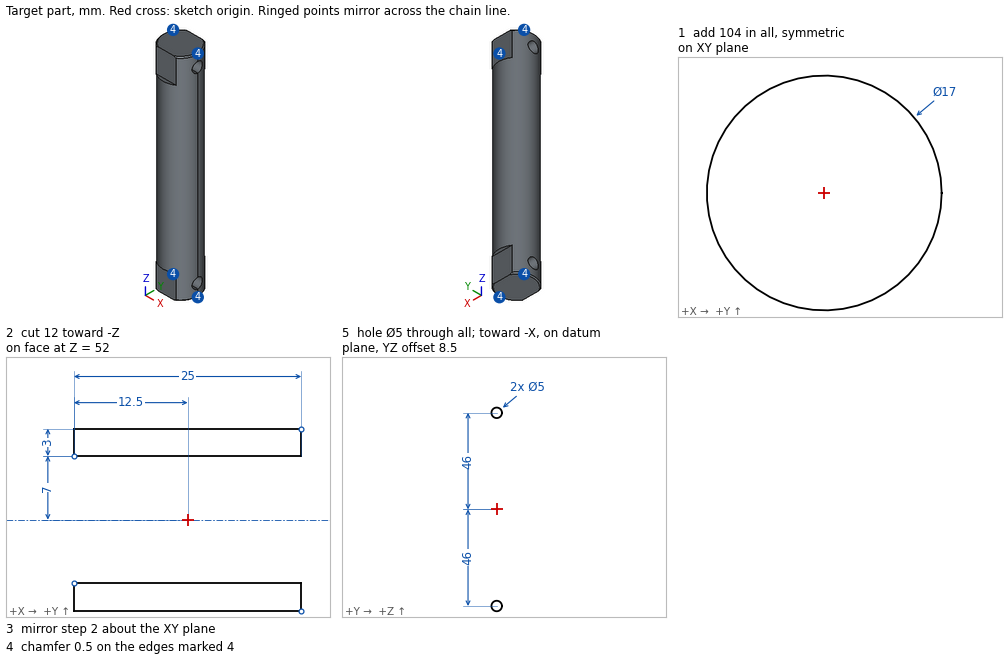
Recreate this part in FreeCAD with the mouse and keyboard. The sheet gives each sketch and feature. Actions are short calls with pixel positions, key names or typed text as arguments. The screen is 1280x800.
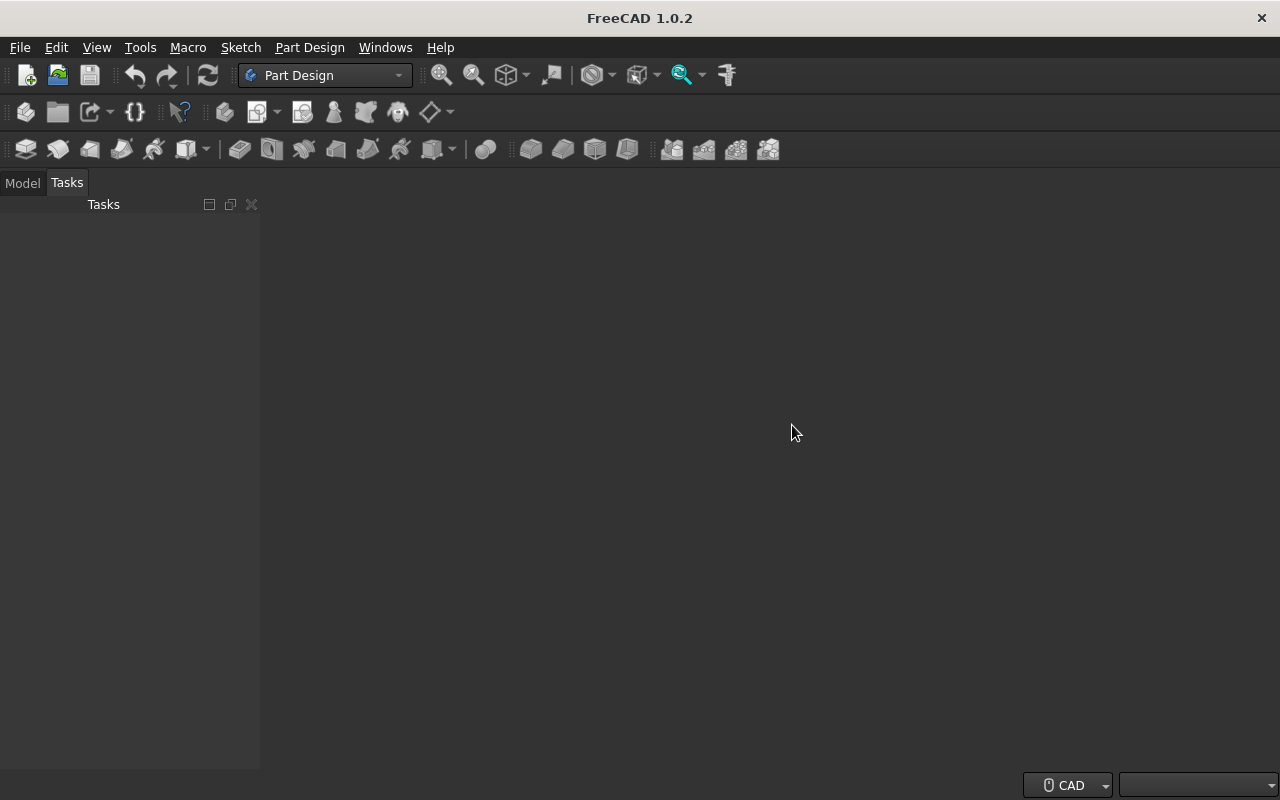
click(26, 76)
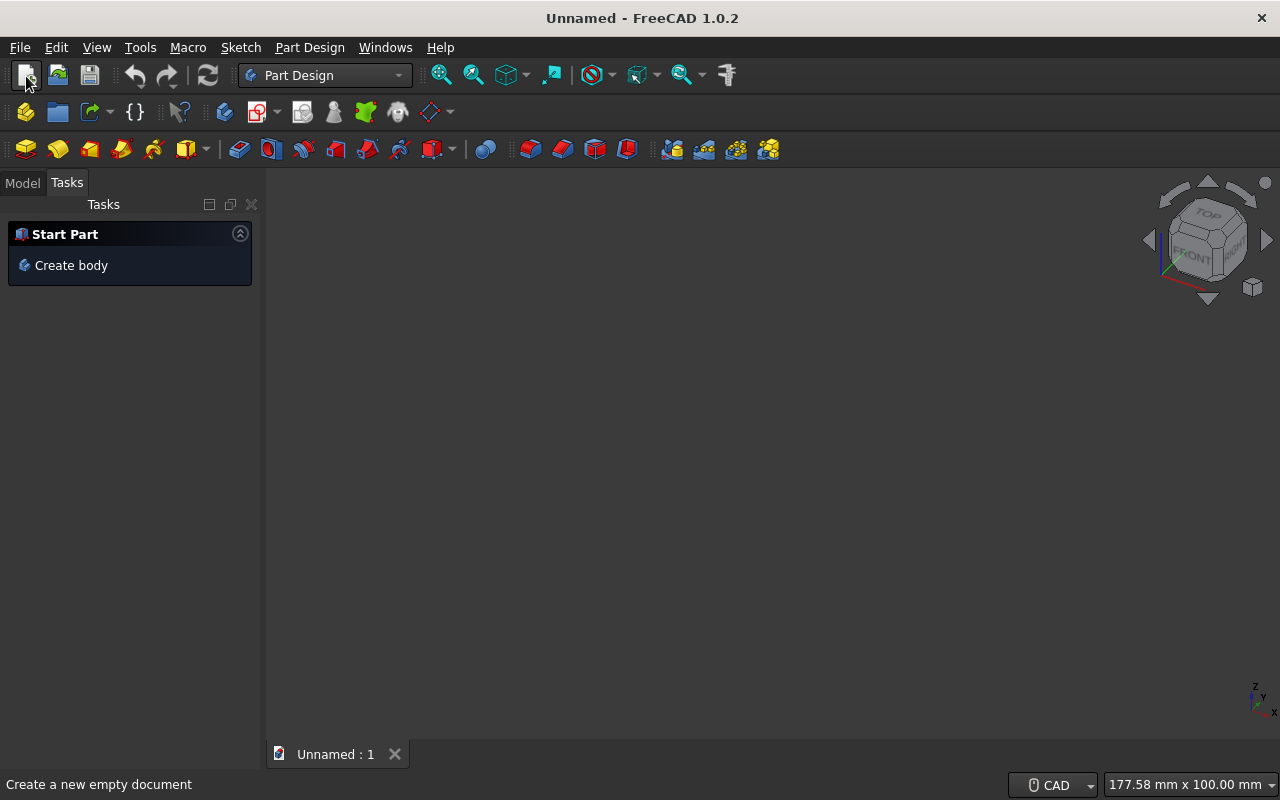
click(258, 112)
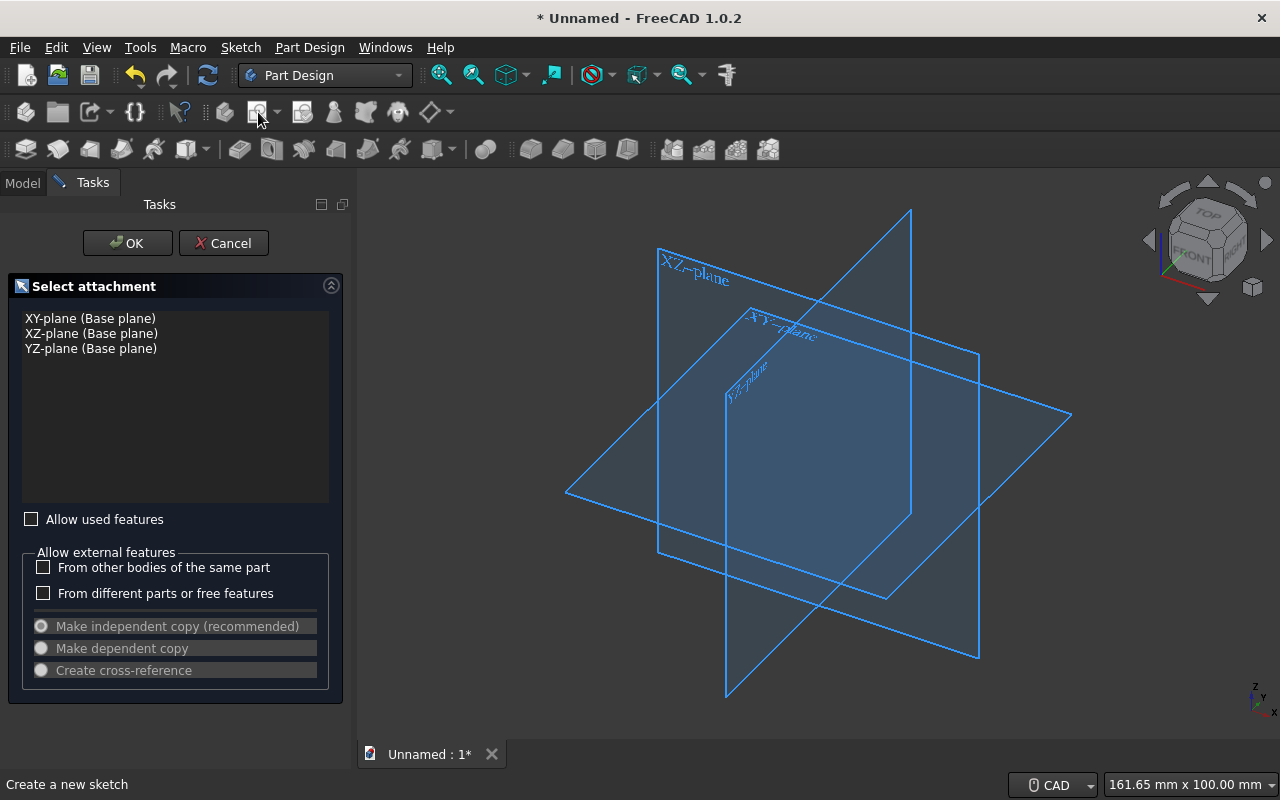
click(82, 318)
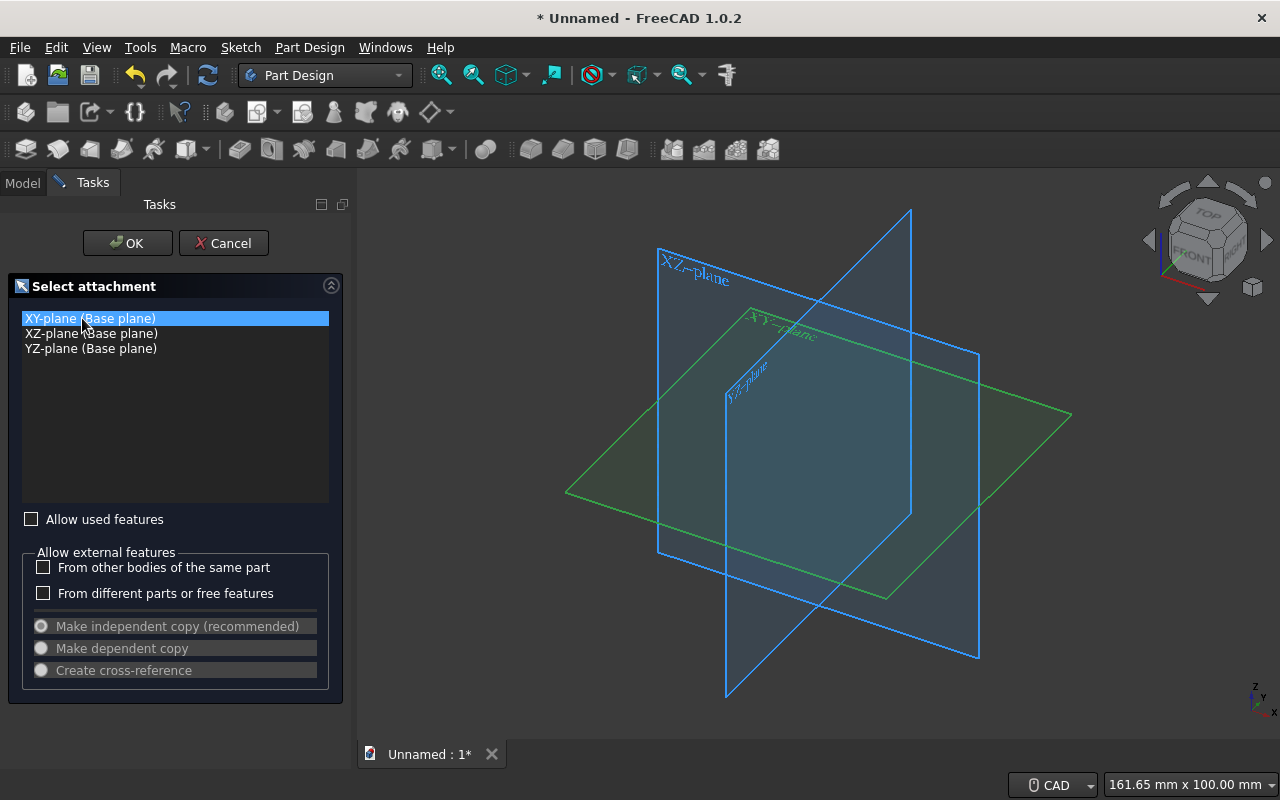
click(128, 243)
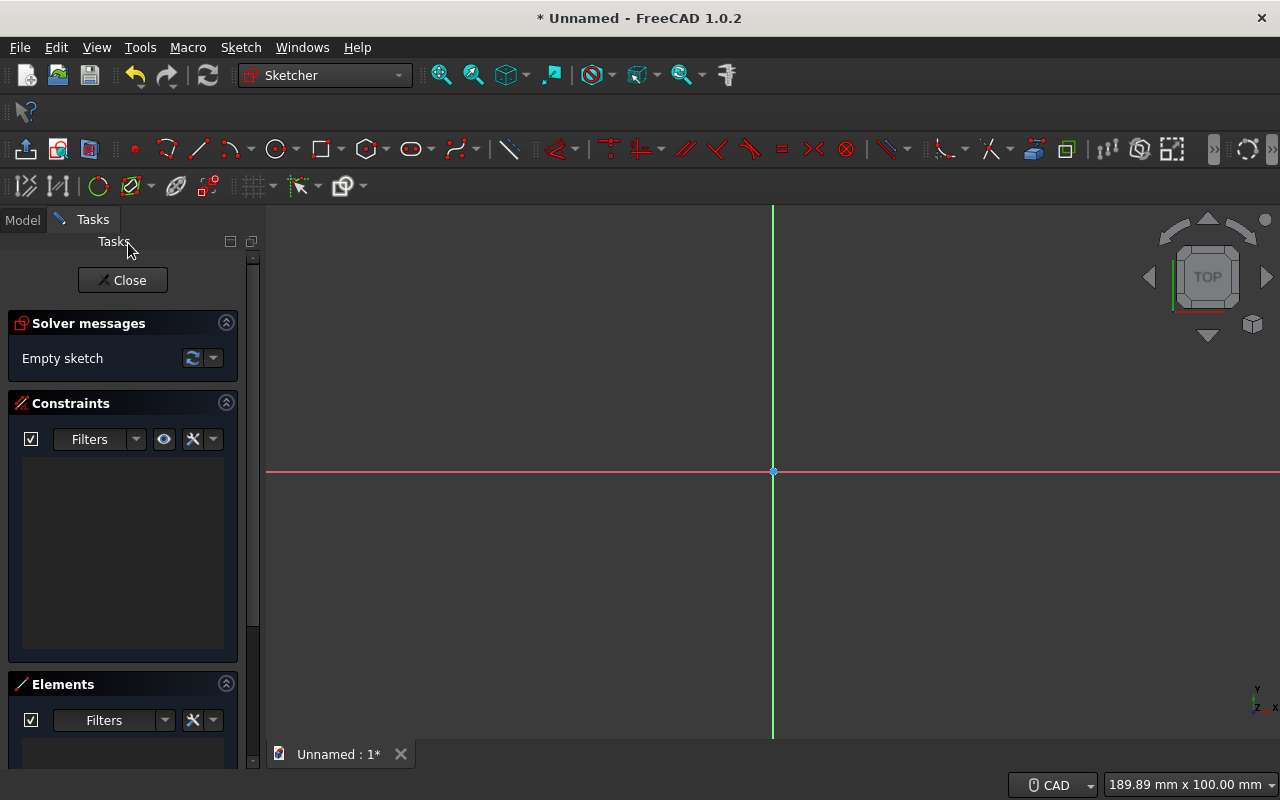
scroll(795, 472, up, 7)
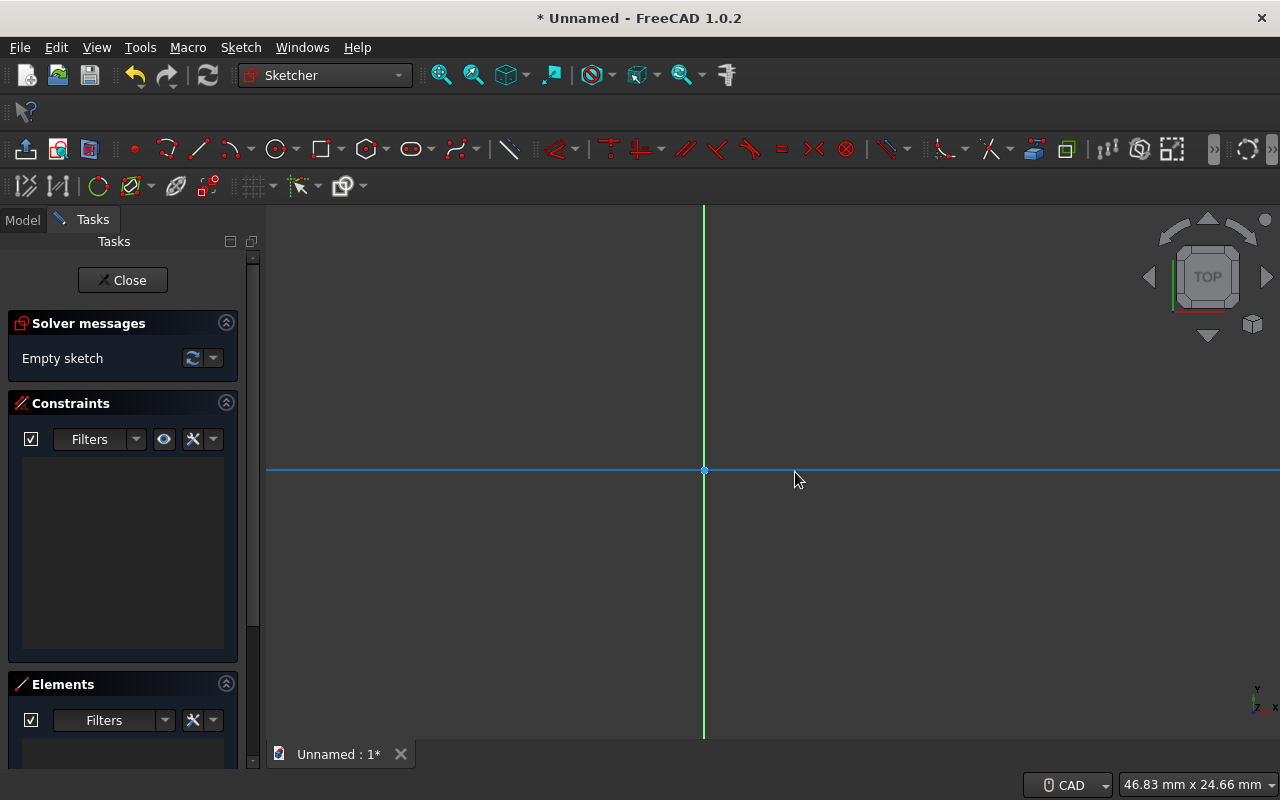
click(276, 150)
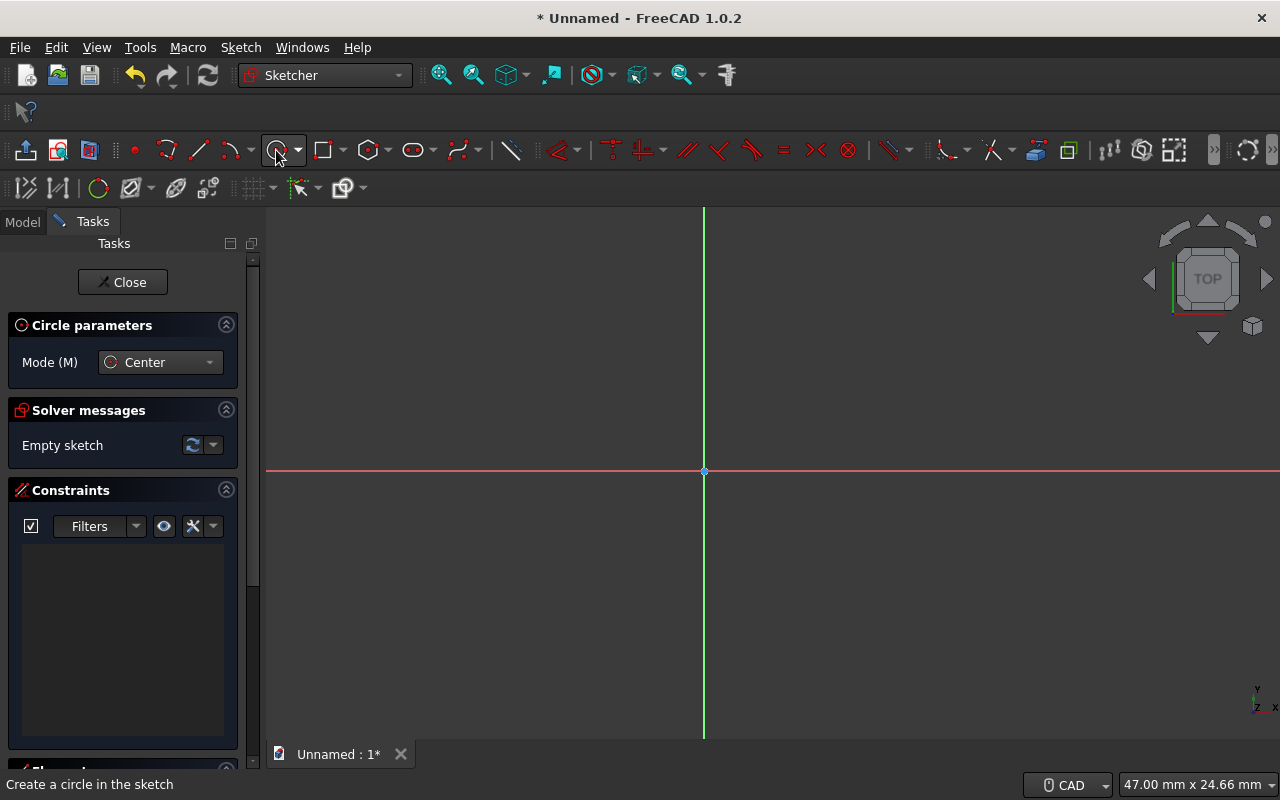
click(704, 471)
click(834, 342)
key(Escape)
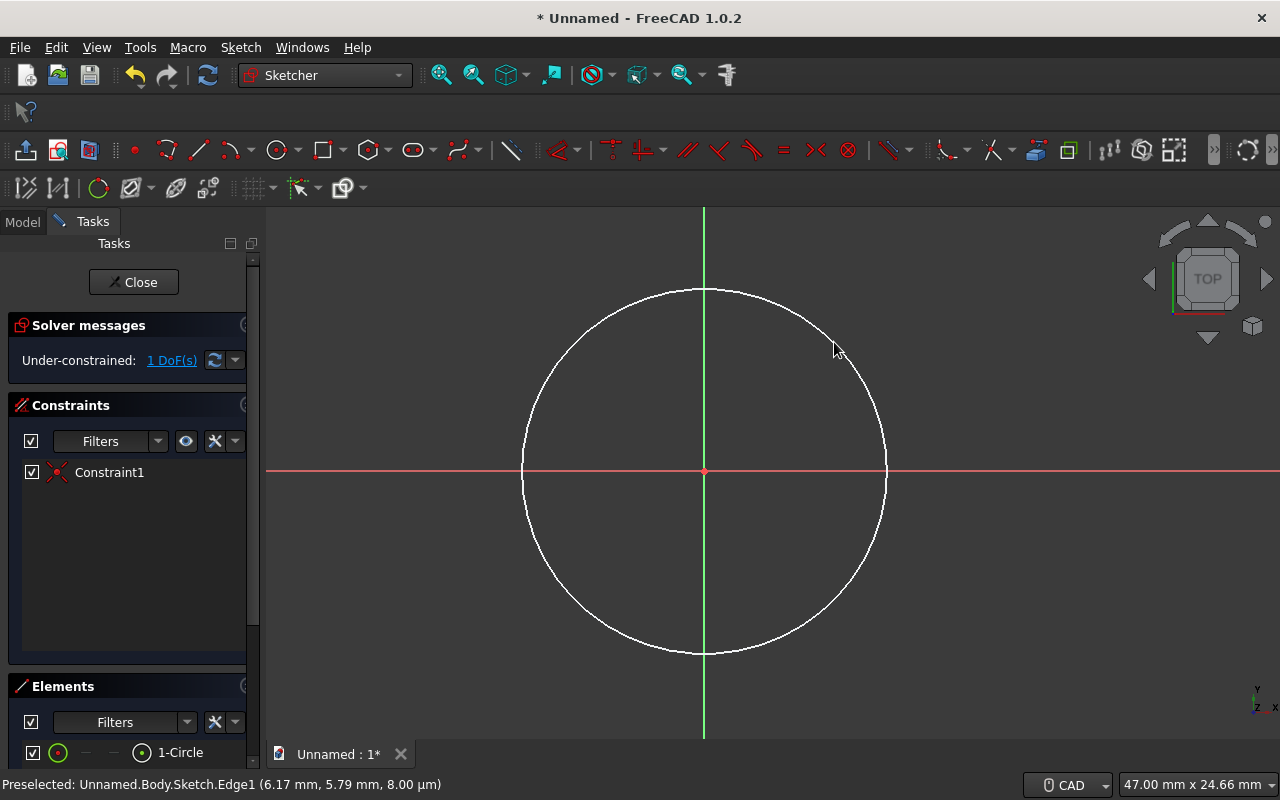
click(558, 150)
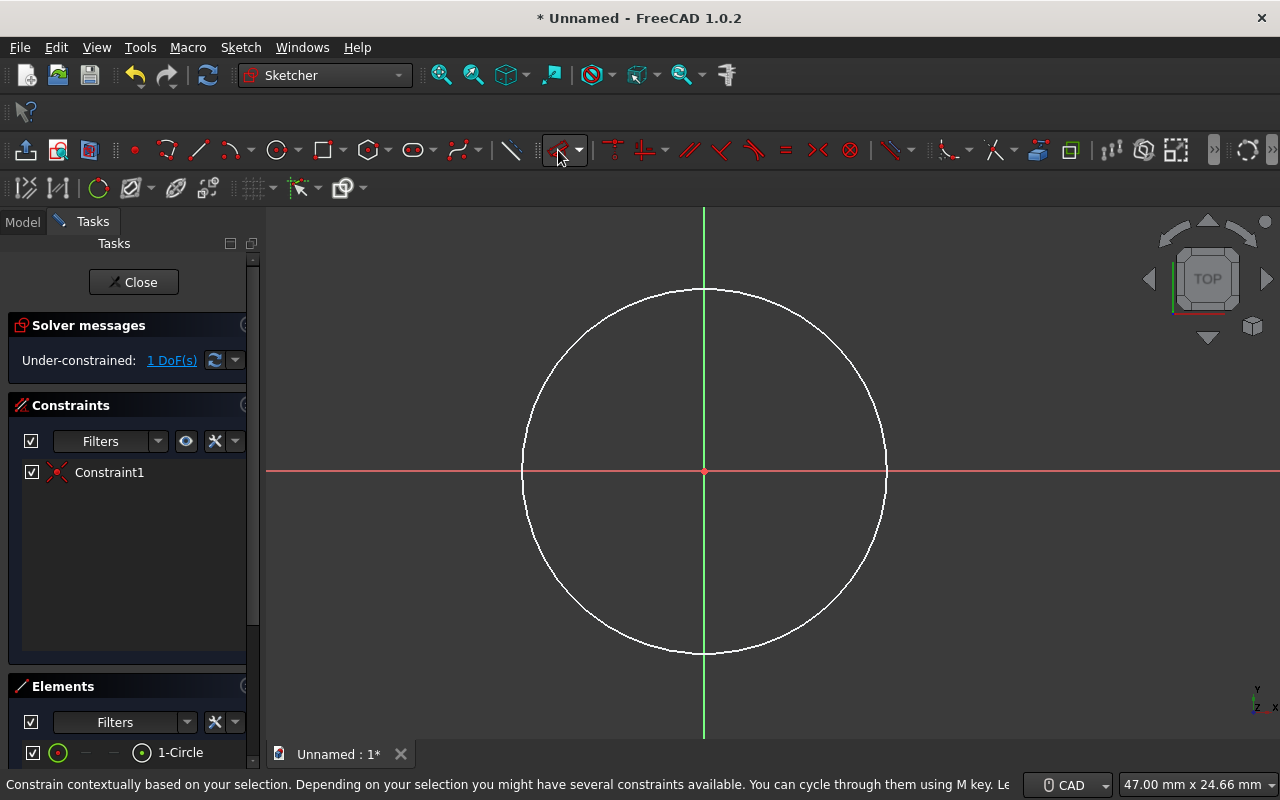
click(833, 342)
click(856, 319)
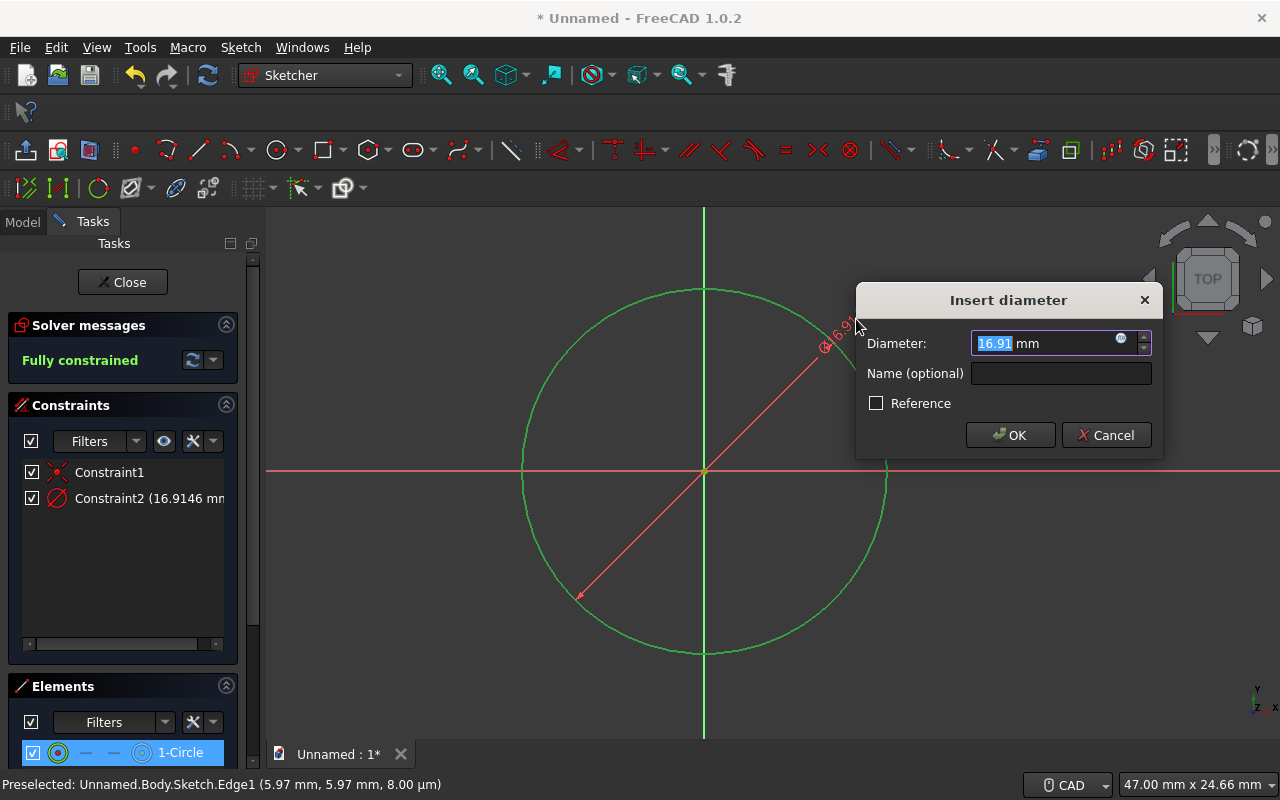
text(17)
key(Return)
key(Escape)